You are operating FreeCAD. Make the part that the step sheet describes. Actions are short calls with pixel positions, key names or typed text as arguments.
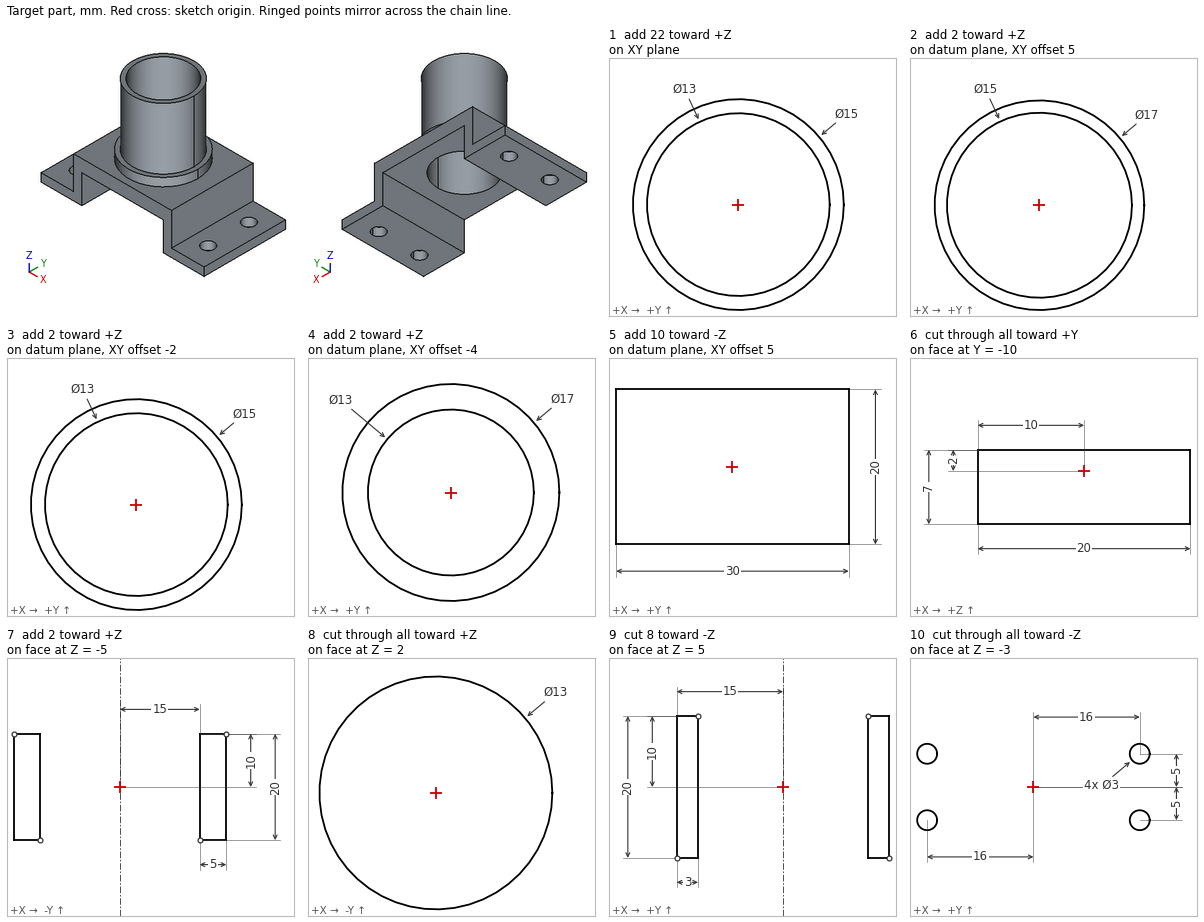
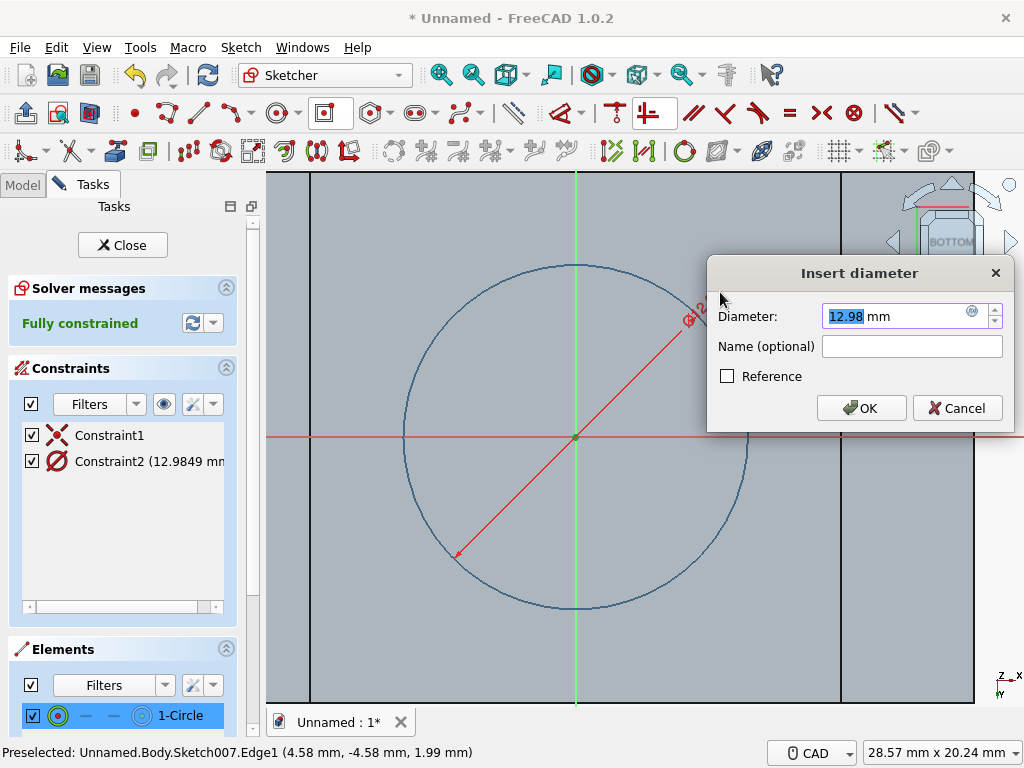
text(13)
key(Return)
key(Escape)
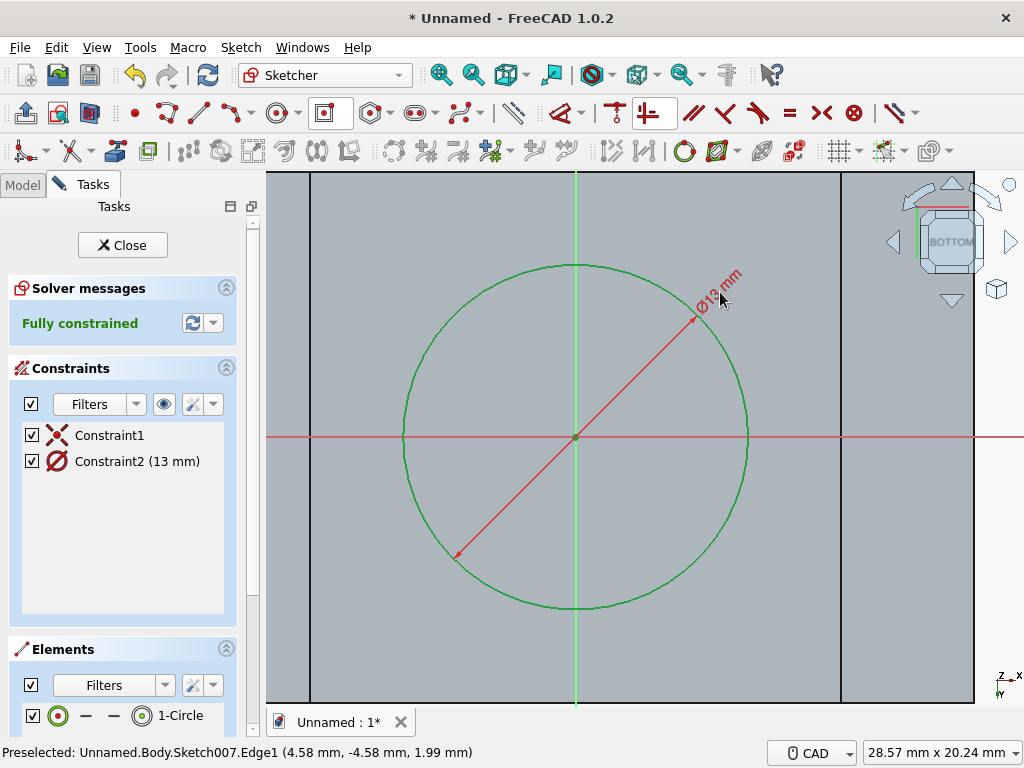
click(123, 245)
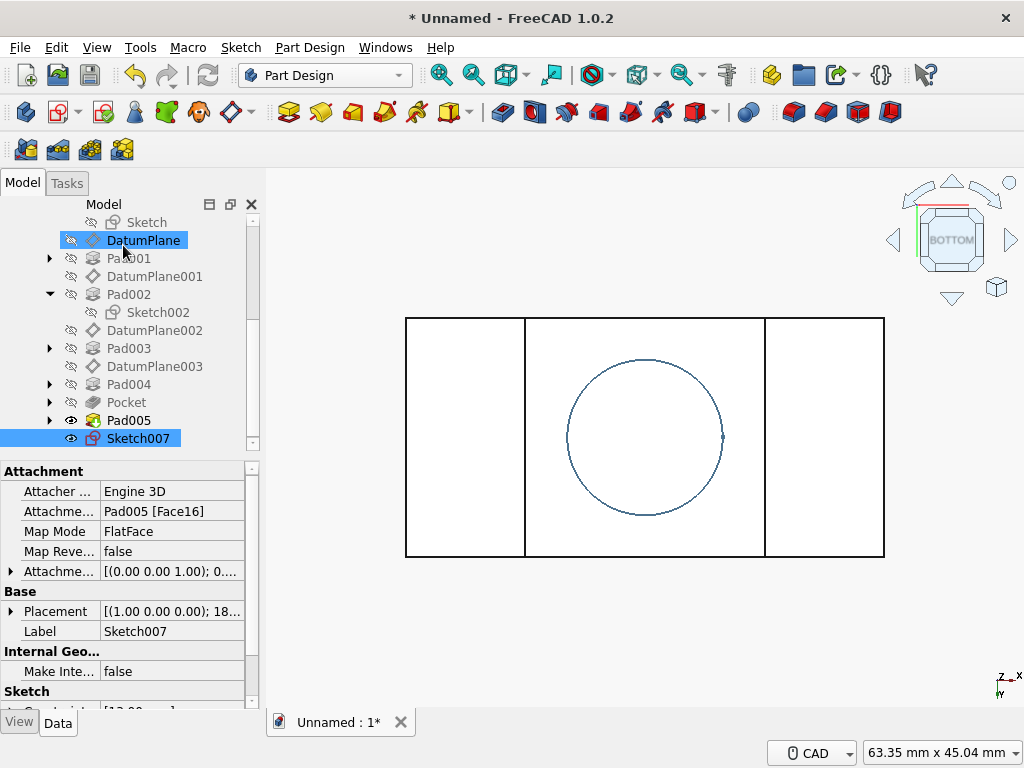
click(504, 112)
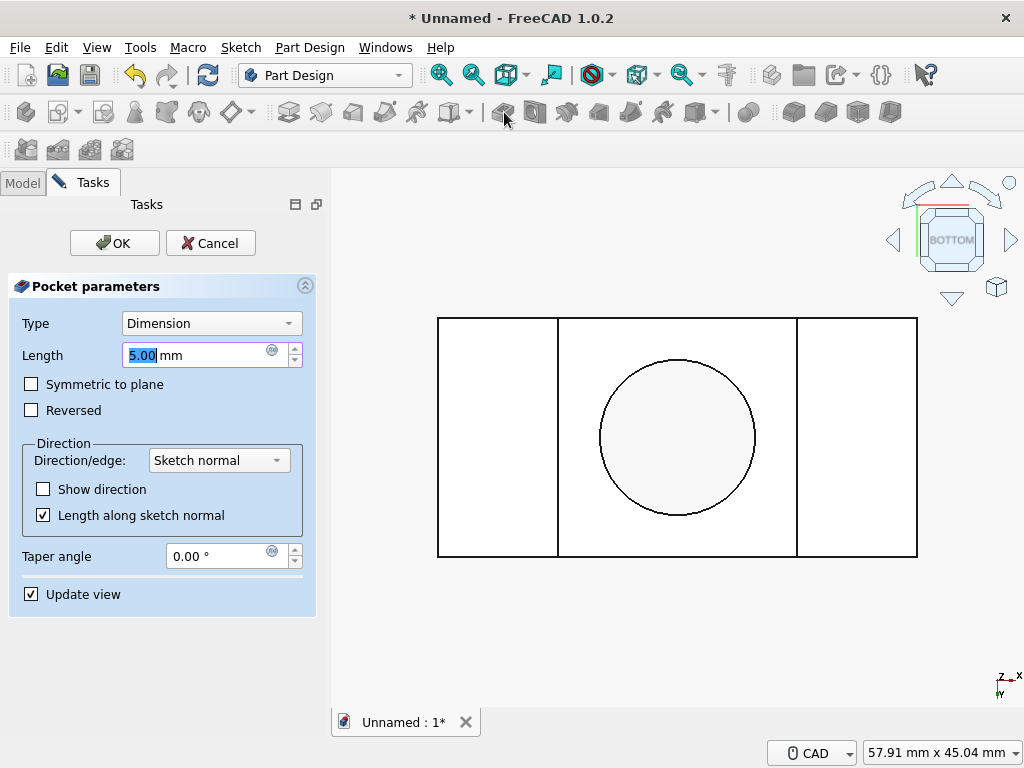
click(212, 324)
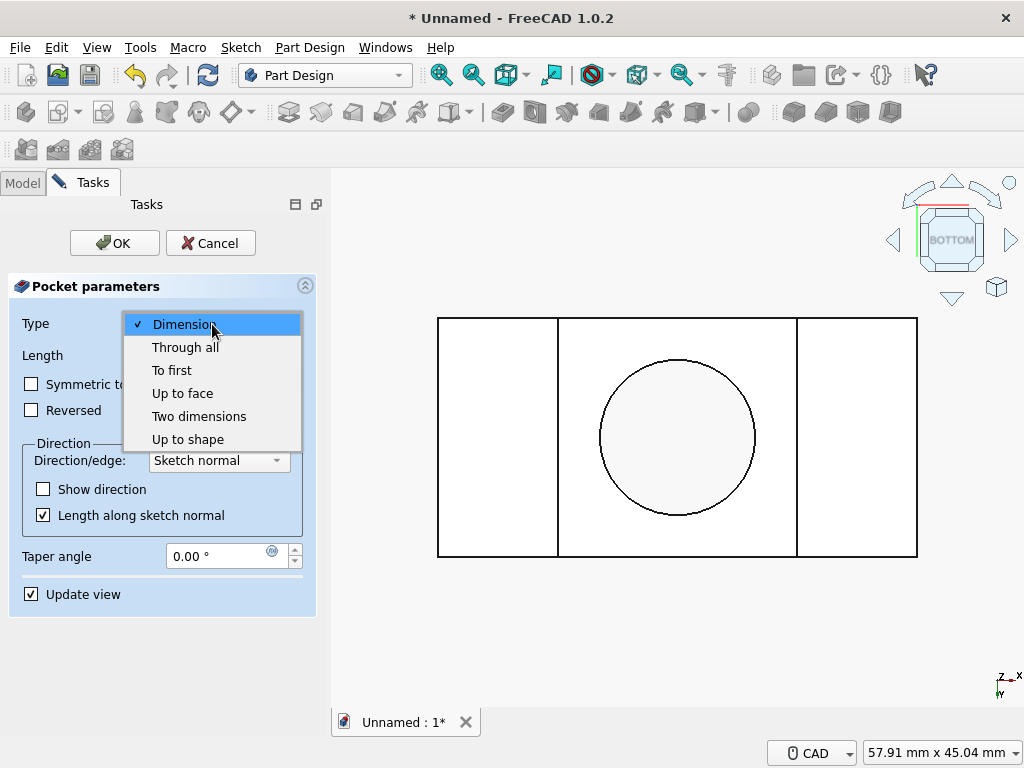
click(212, 348)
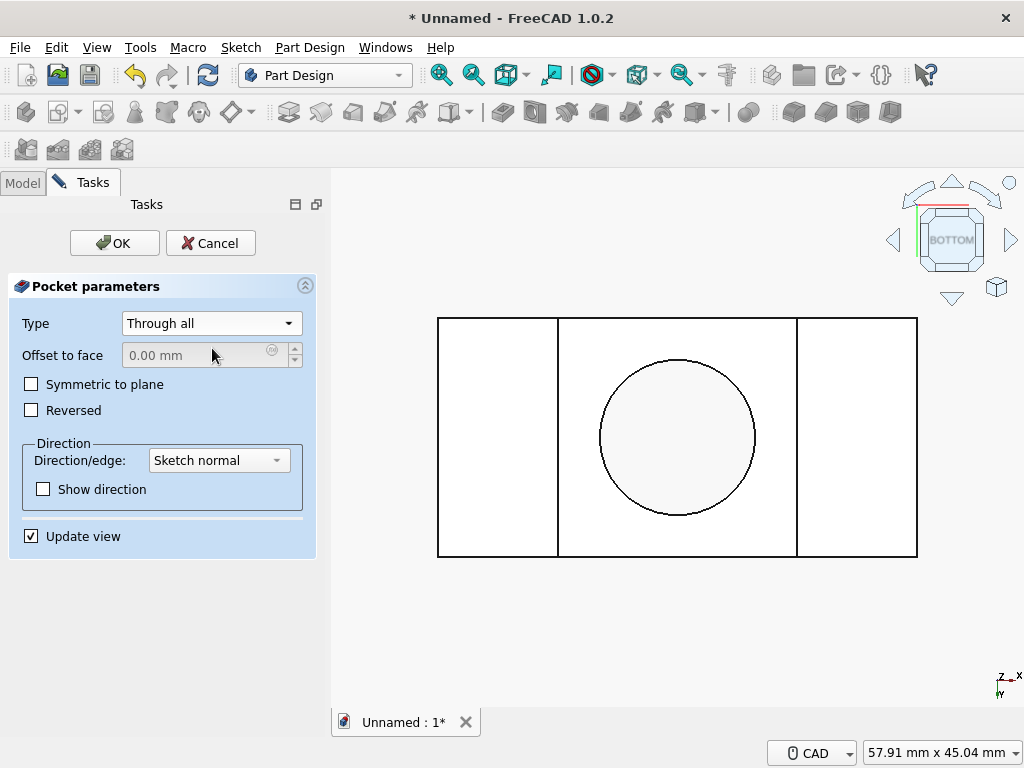
click(115, 243)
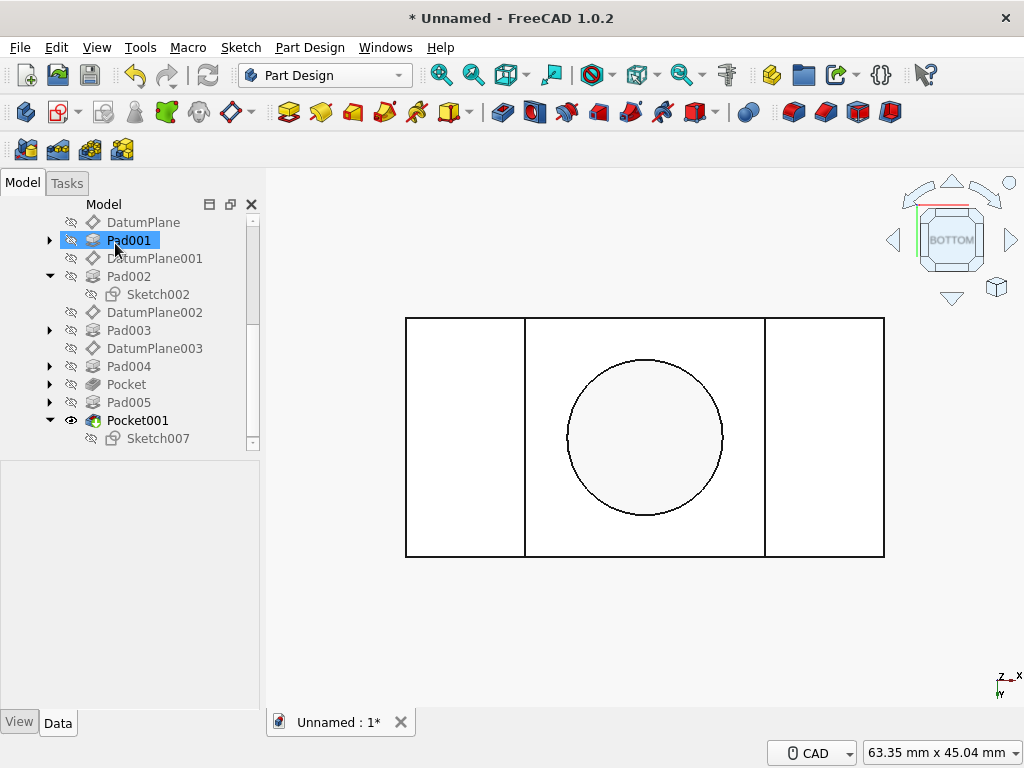
key(0)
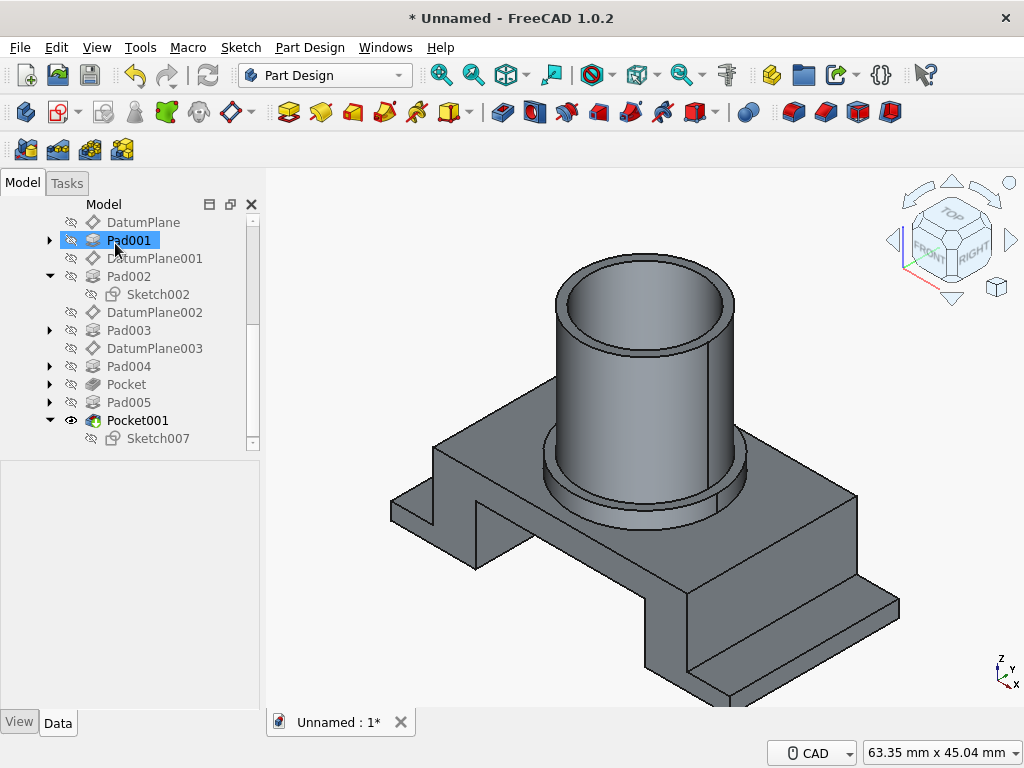
click(442, 76)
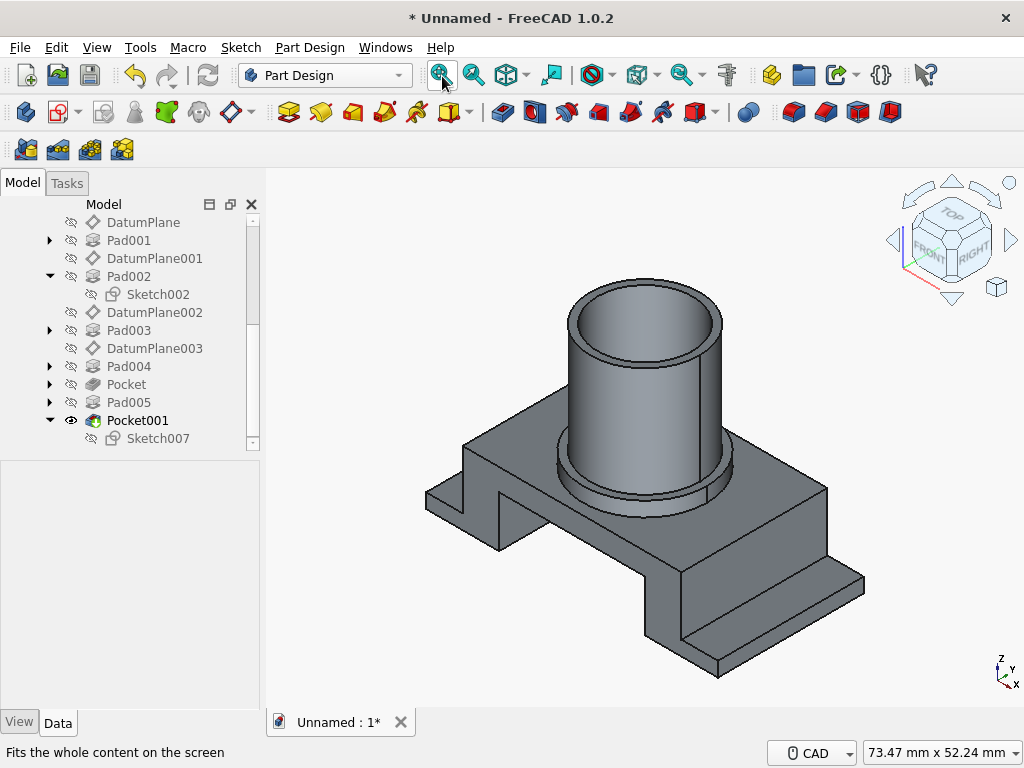
click(780, 496)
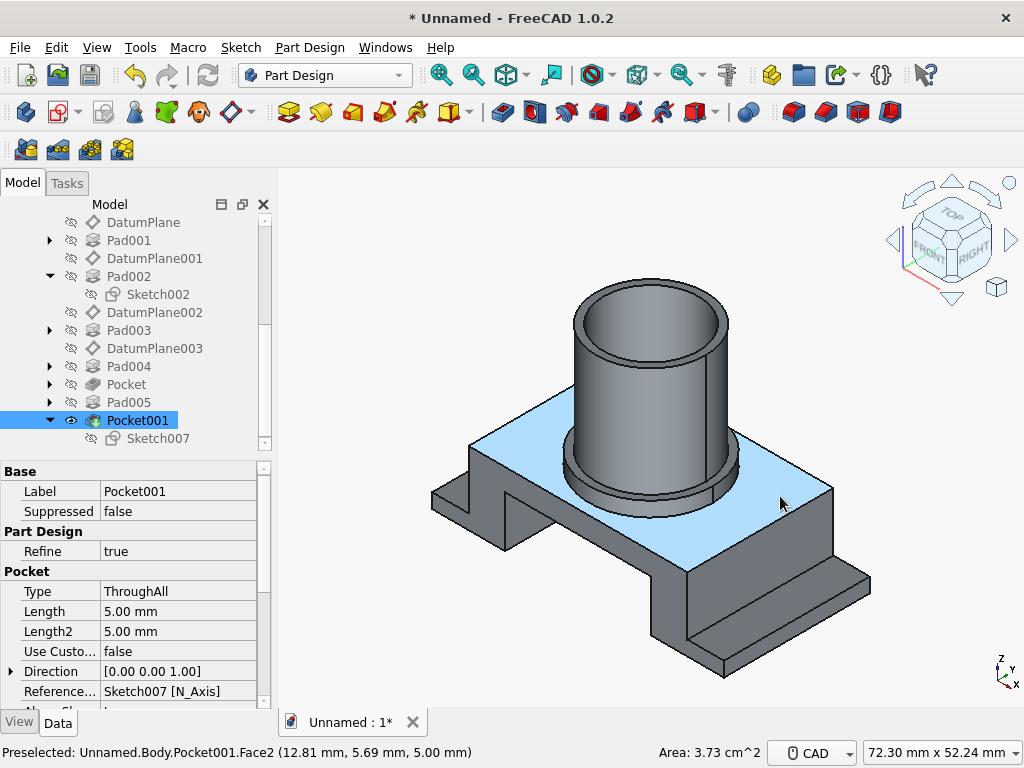
click(58, 112)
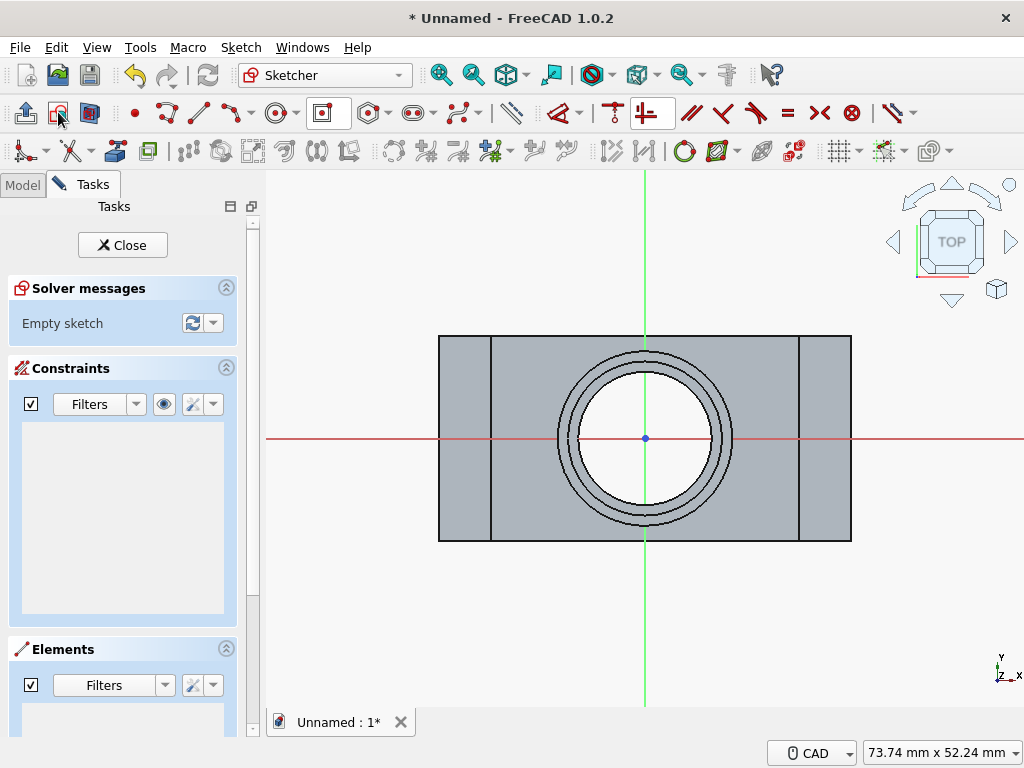
click(90, 114)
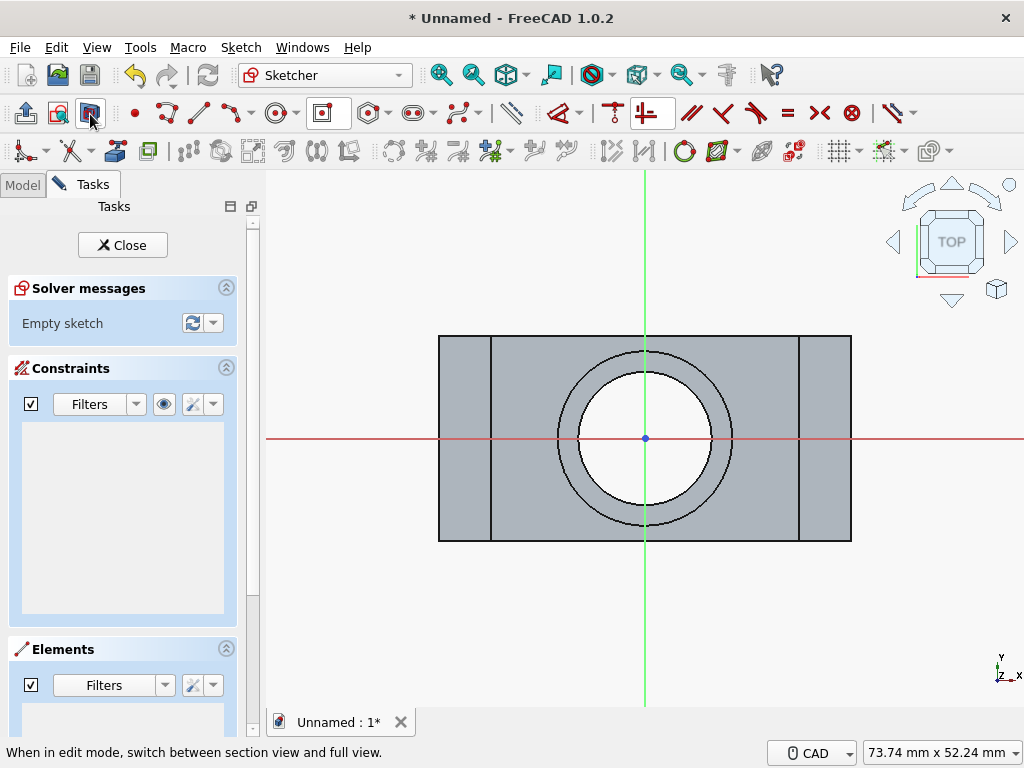
key(g)
key(r)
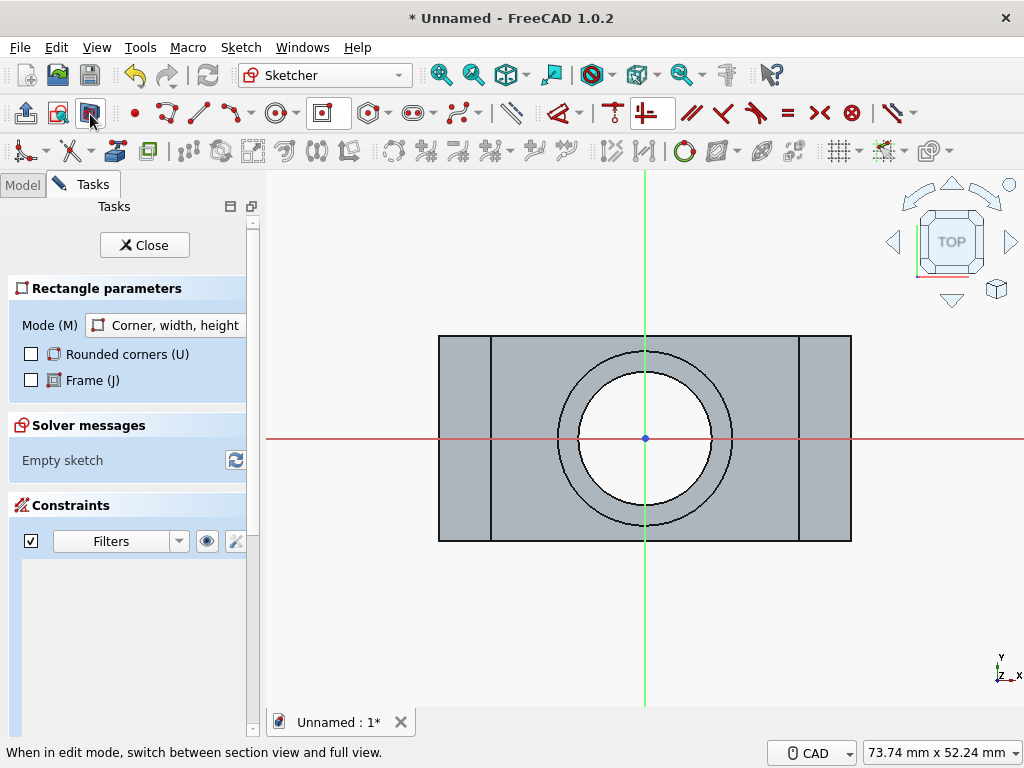
click(491, 336)
click(522, 541)